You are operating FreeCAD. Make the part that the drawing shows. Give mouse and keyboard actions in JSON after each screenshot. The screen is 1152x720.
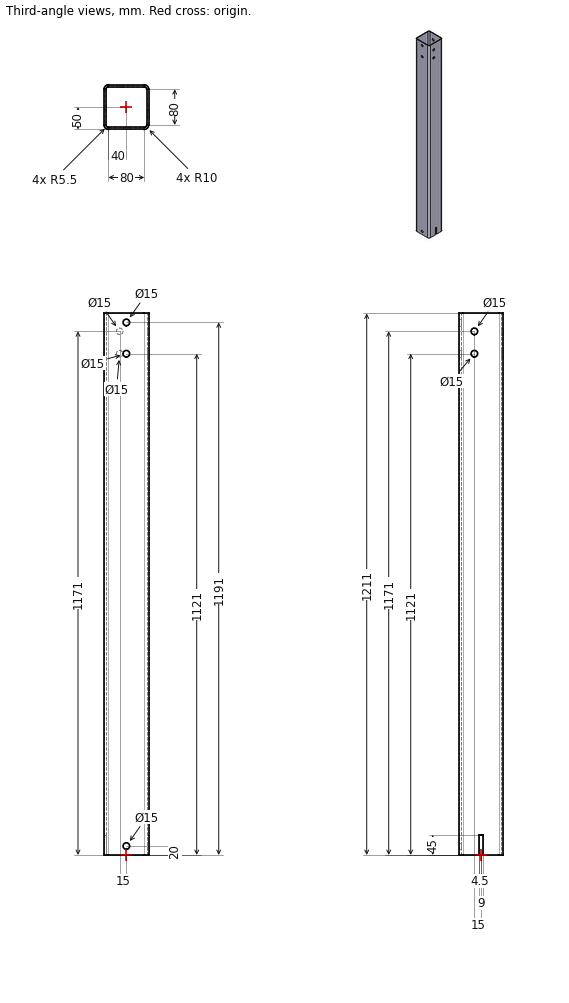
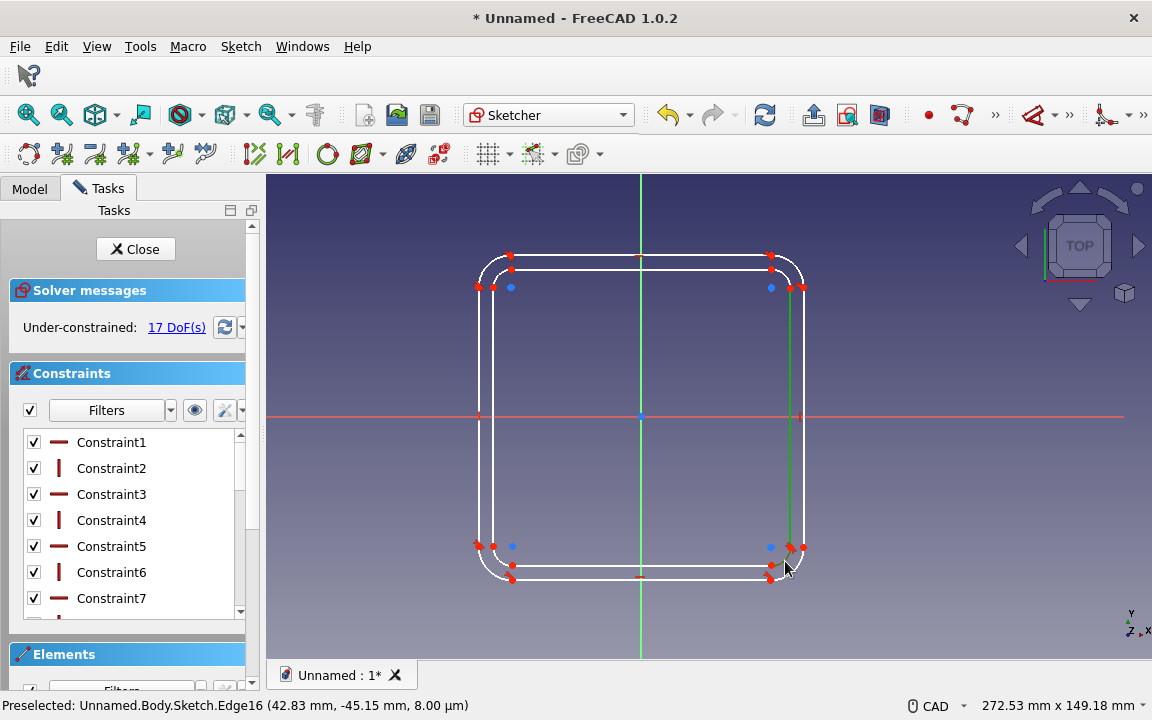
{"action": "key", "text": "t"}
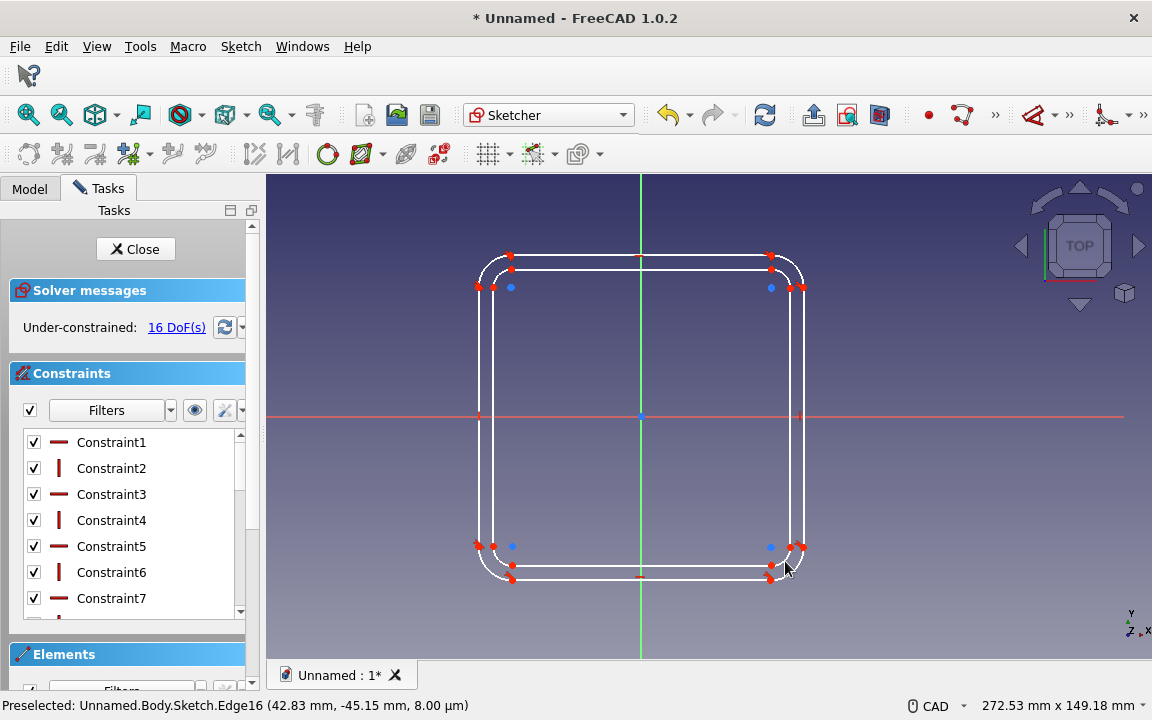
{"action": "left_click", "coordinate": [482, 562]}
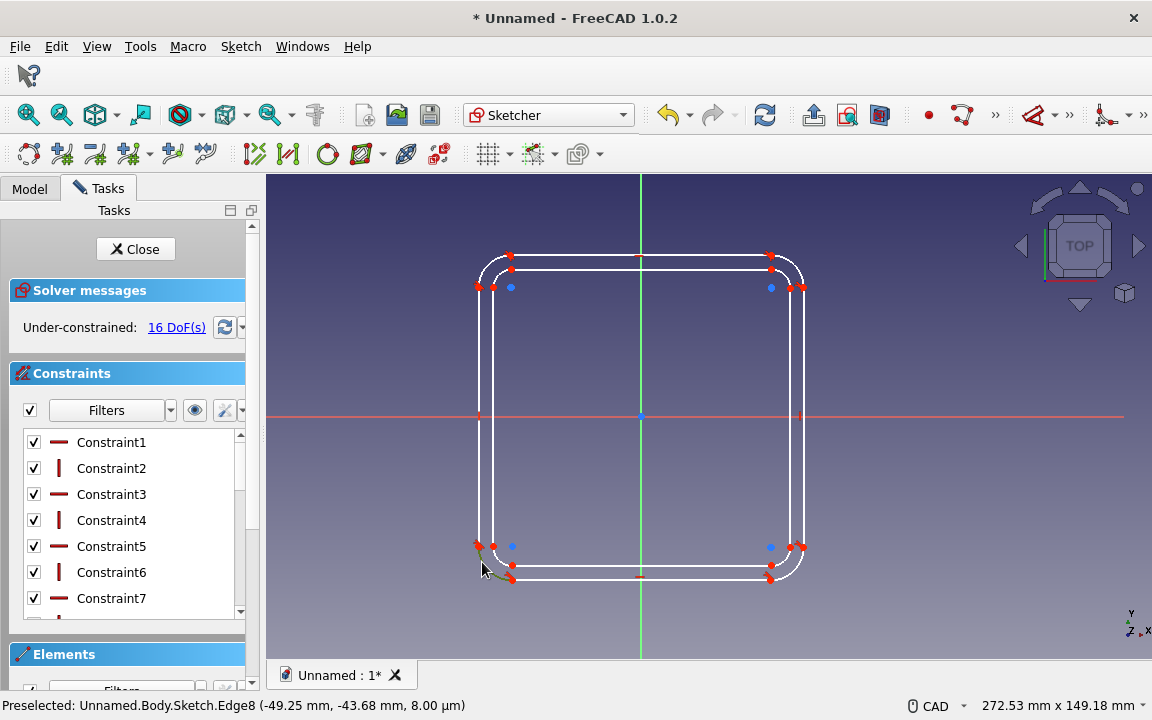
{"action": "left_click", "coordinate": [499, 560]}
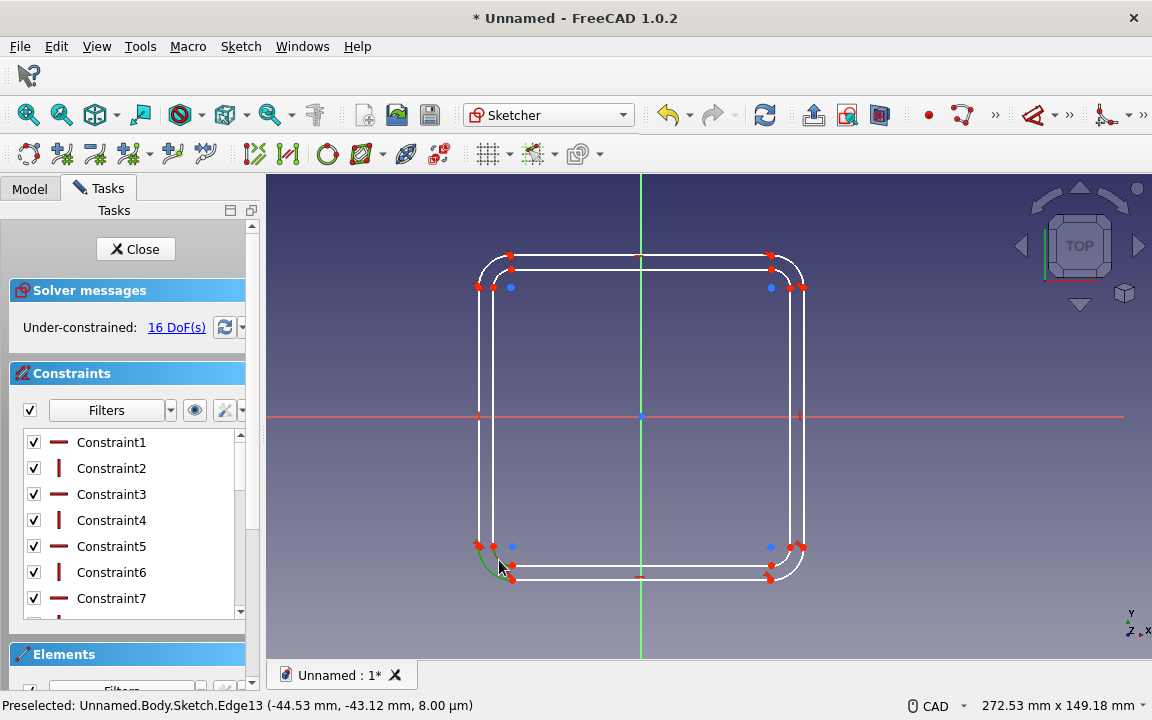
{"action": "key", "text": "c"}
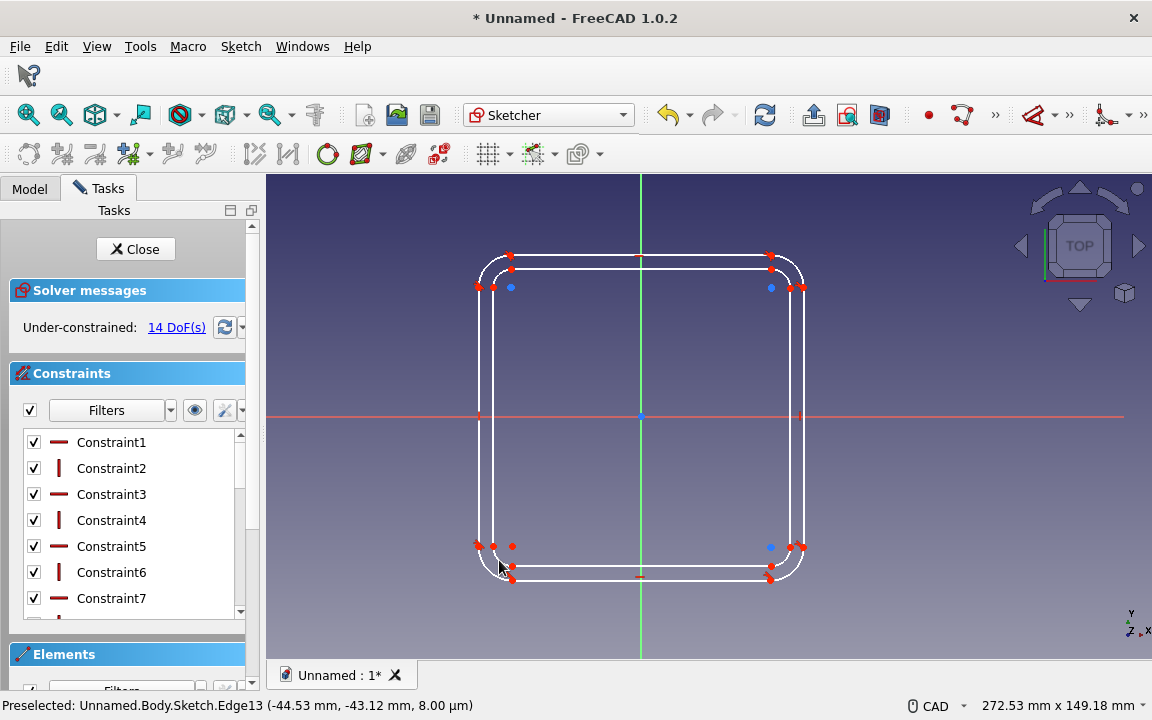
{"action": "left_click", "coordinate": [496, 259]}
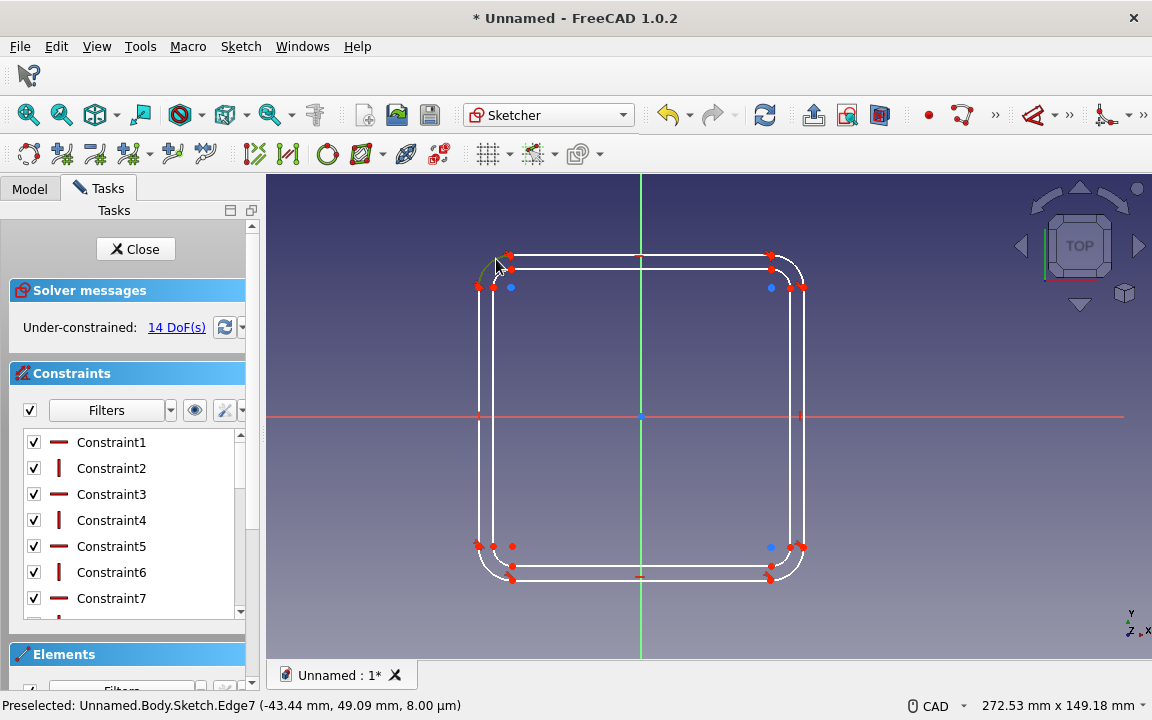
{"action": "left_click", "coordinate": [499, 275]}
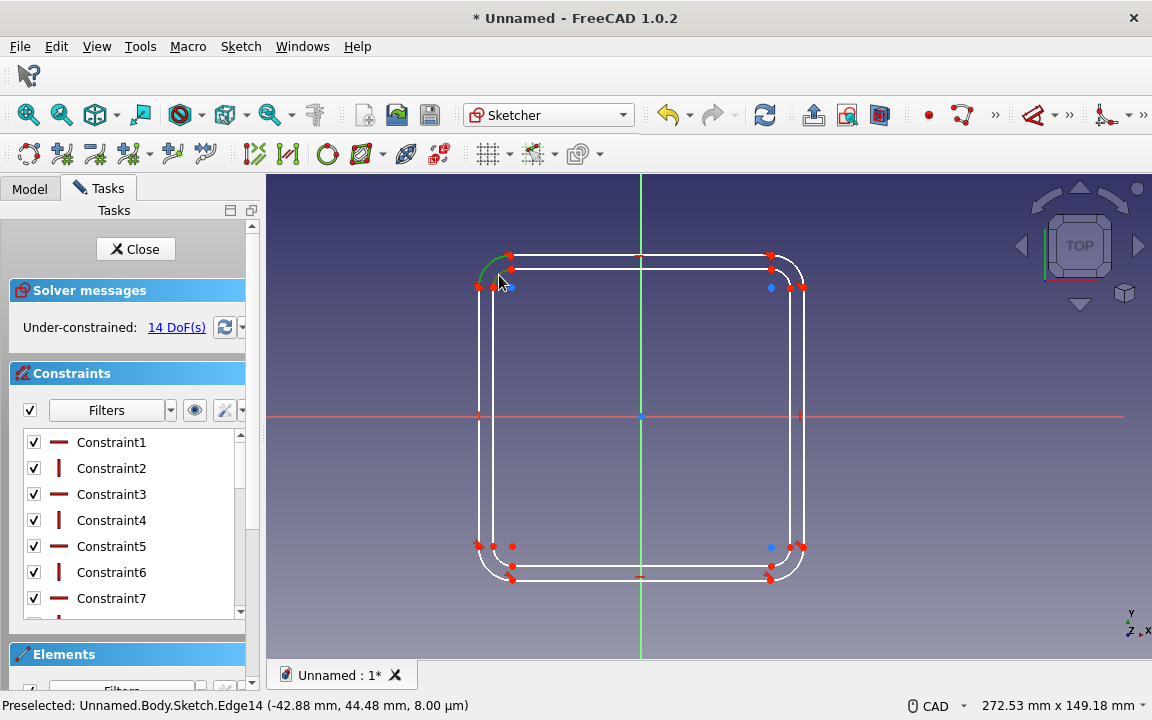
{"action": "key", "text": "c"}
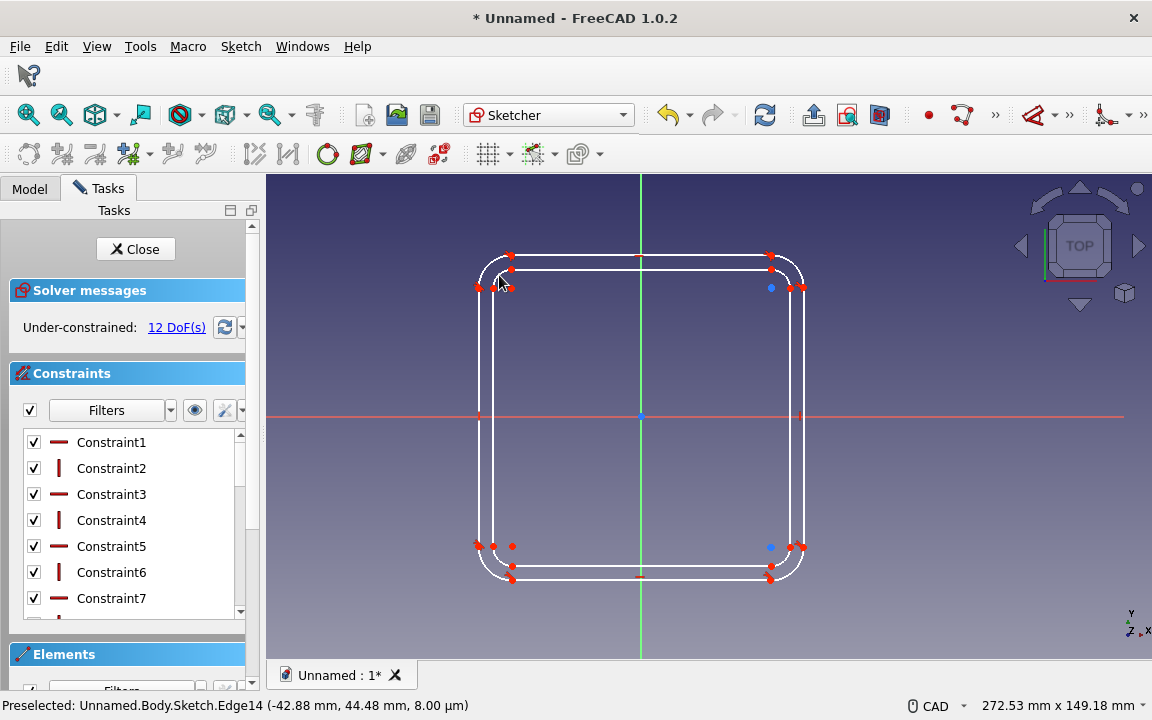
{"action": "left_click", "coordinate": [800, 273]}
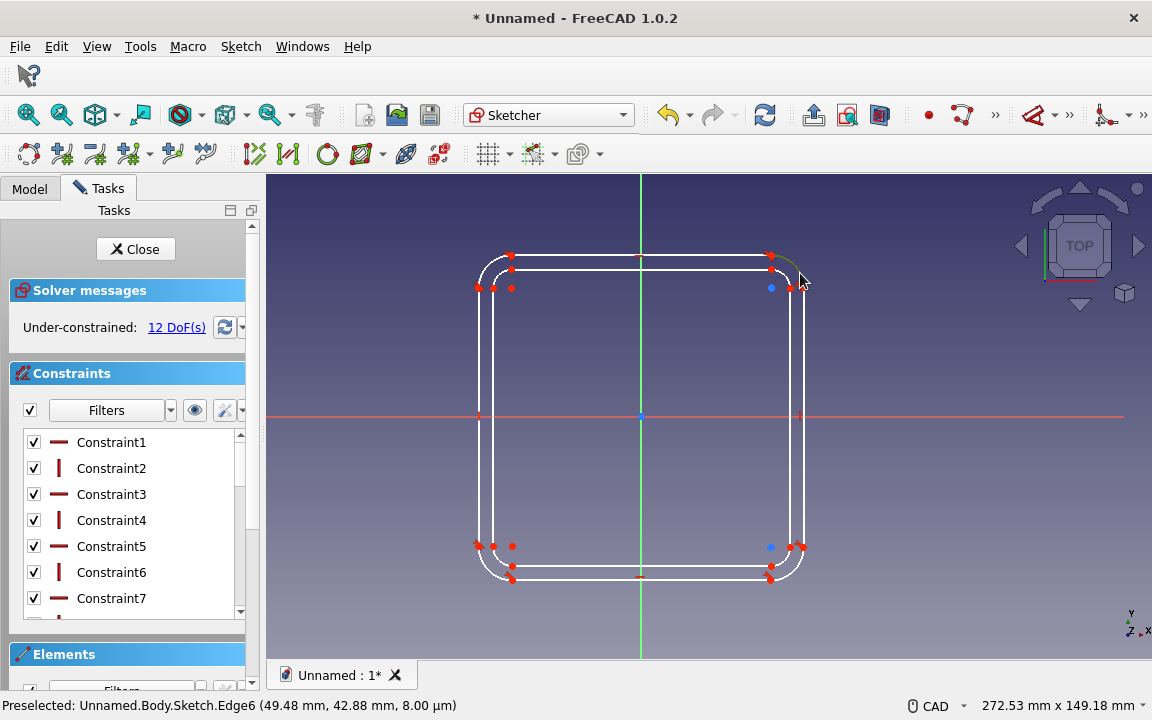
{"action": "left_click", "coordinate": [785, 275]}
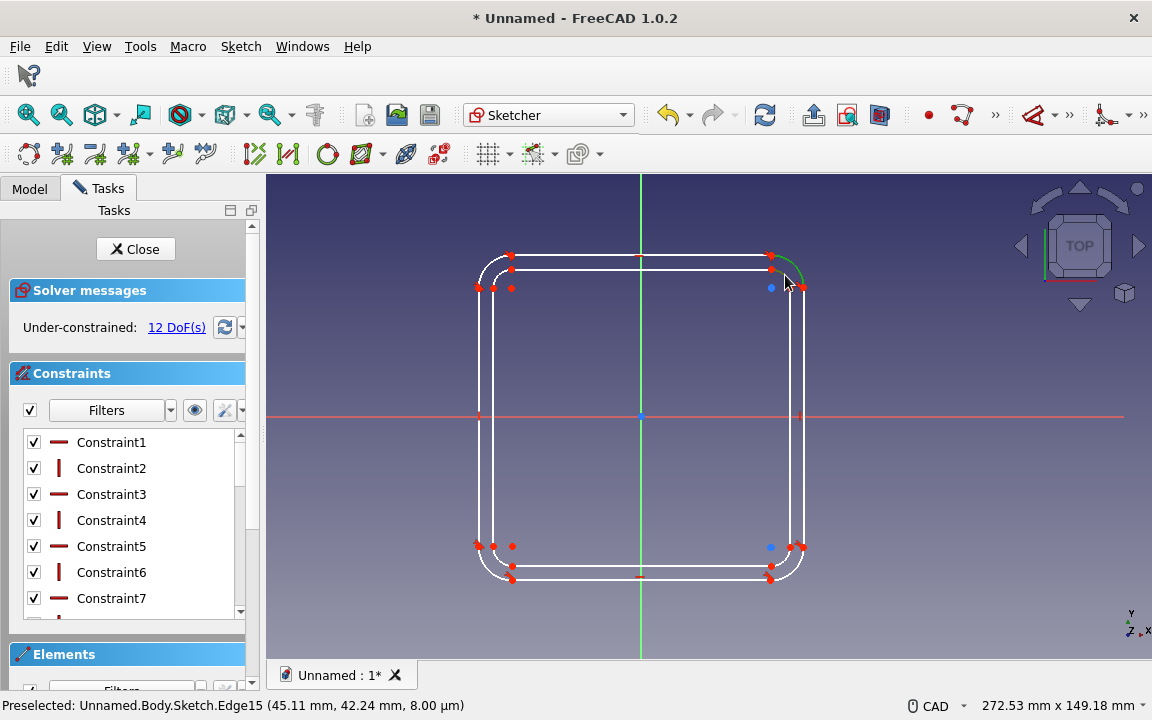
{"action": "key", "text": "c"}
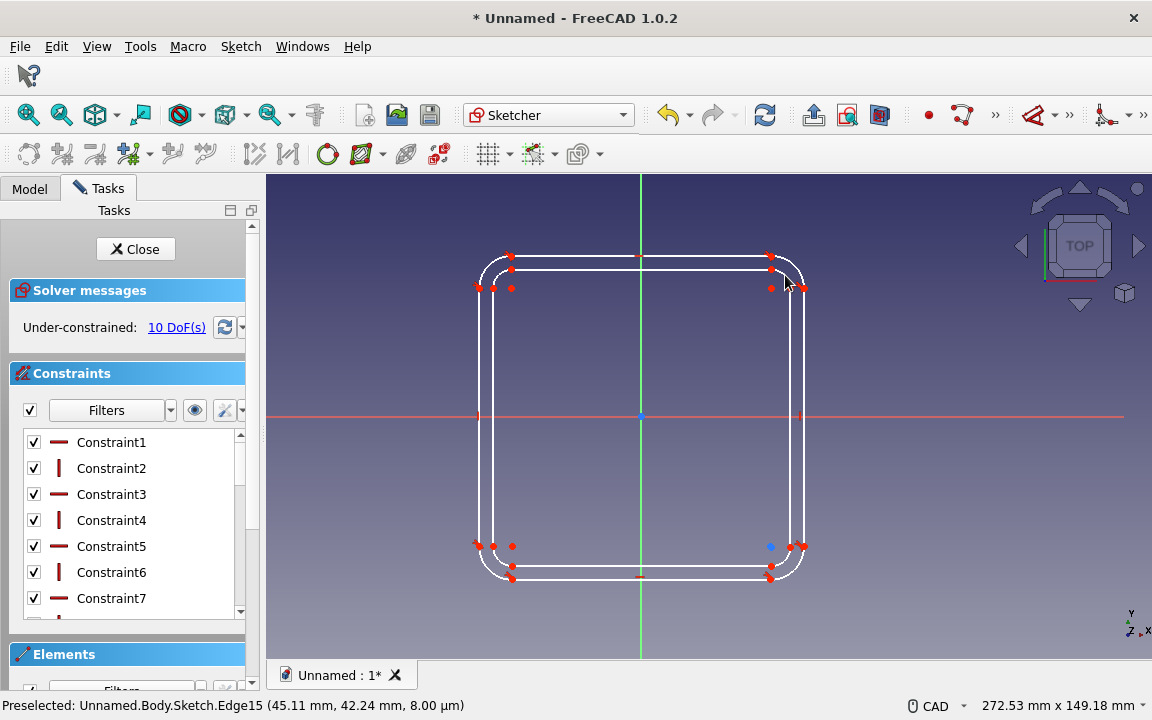
{"action": "left_click", "coordinate": [786, 576]}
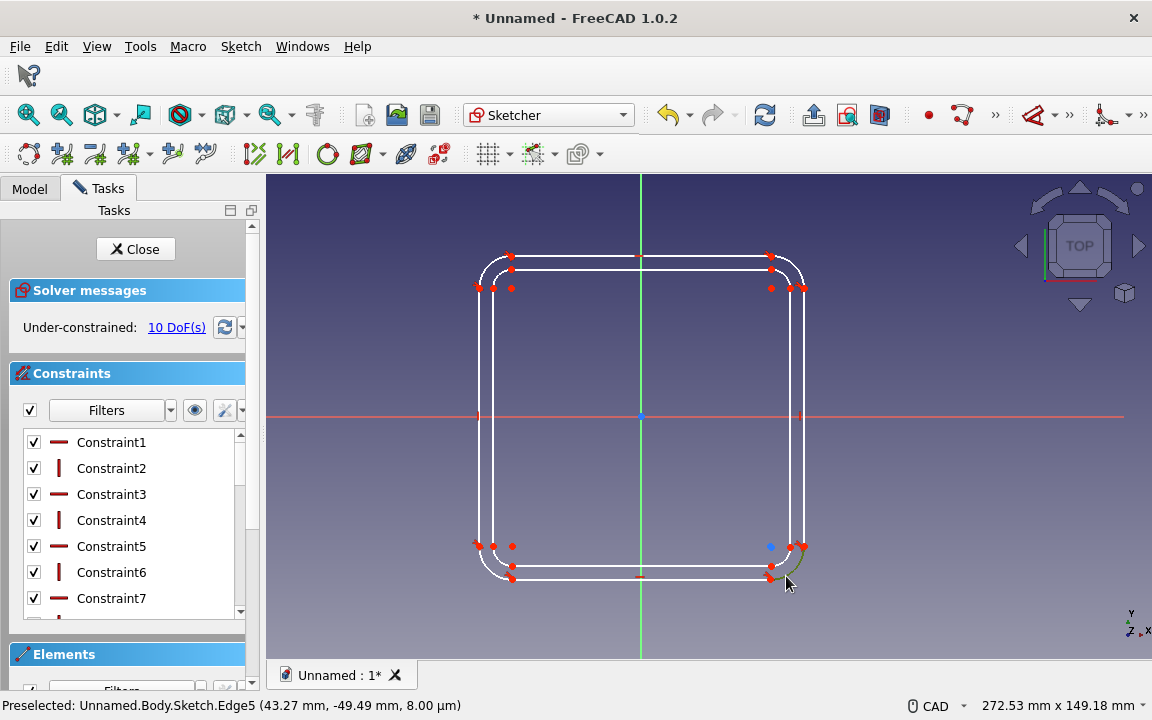
{"action": "left_click", "coordinate": [801, 274]}